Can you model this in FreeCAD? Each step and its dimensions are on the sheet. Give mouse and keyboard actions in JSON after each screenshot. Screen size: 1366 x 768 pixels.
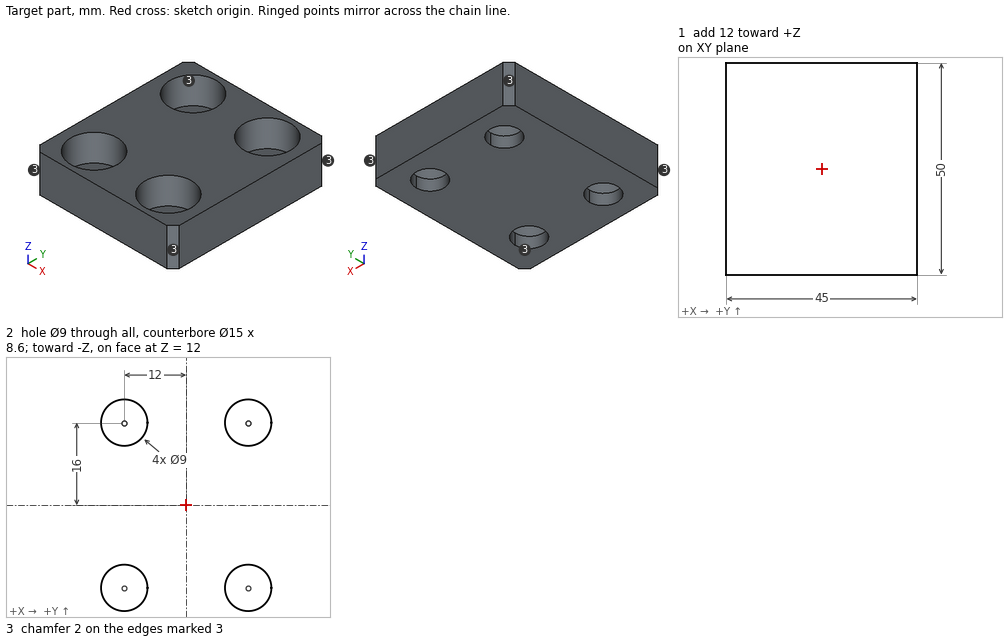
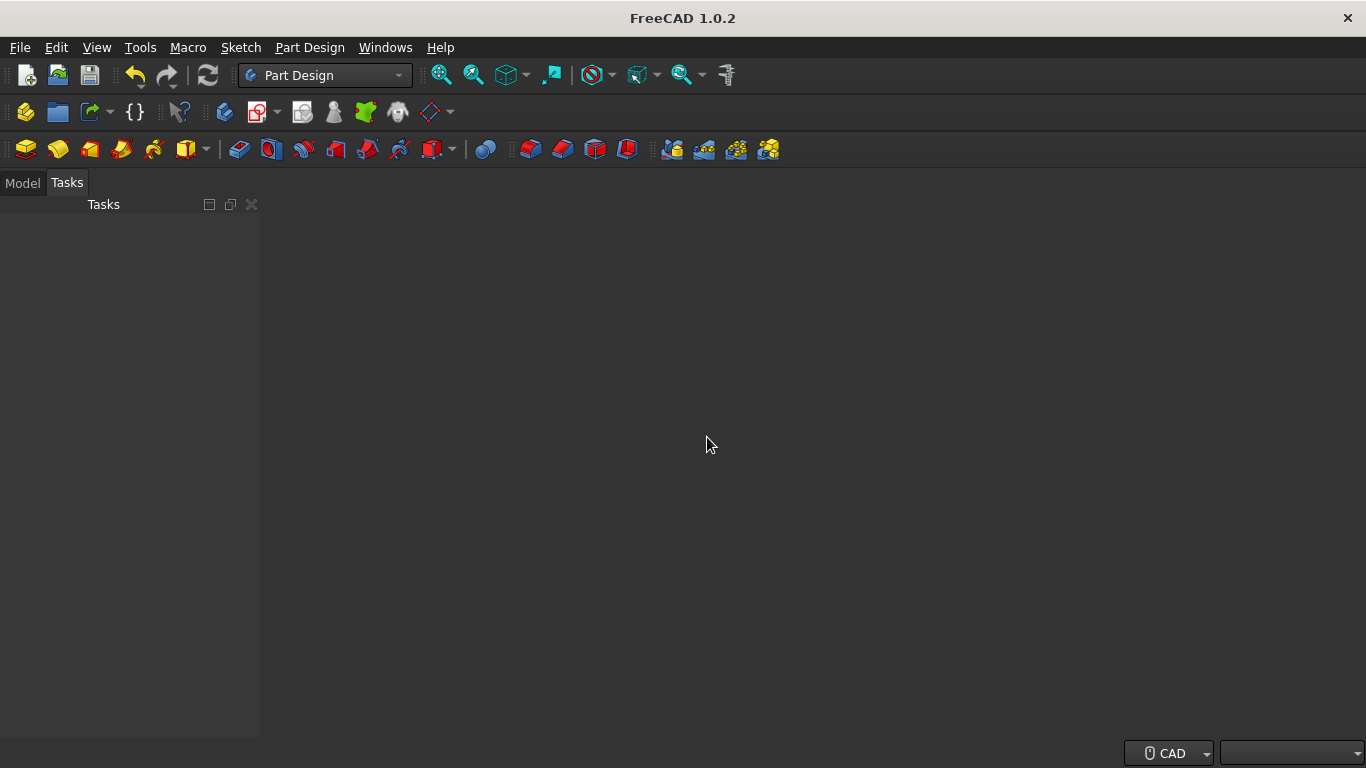
{"action": "left_click", "coordinate": [26, 76]}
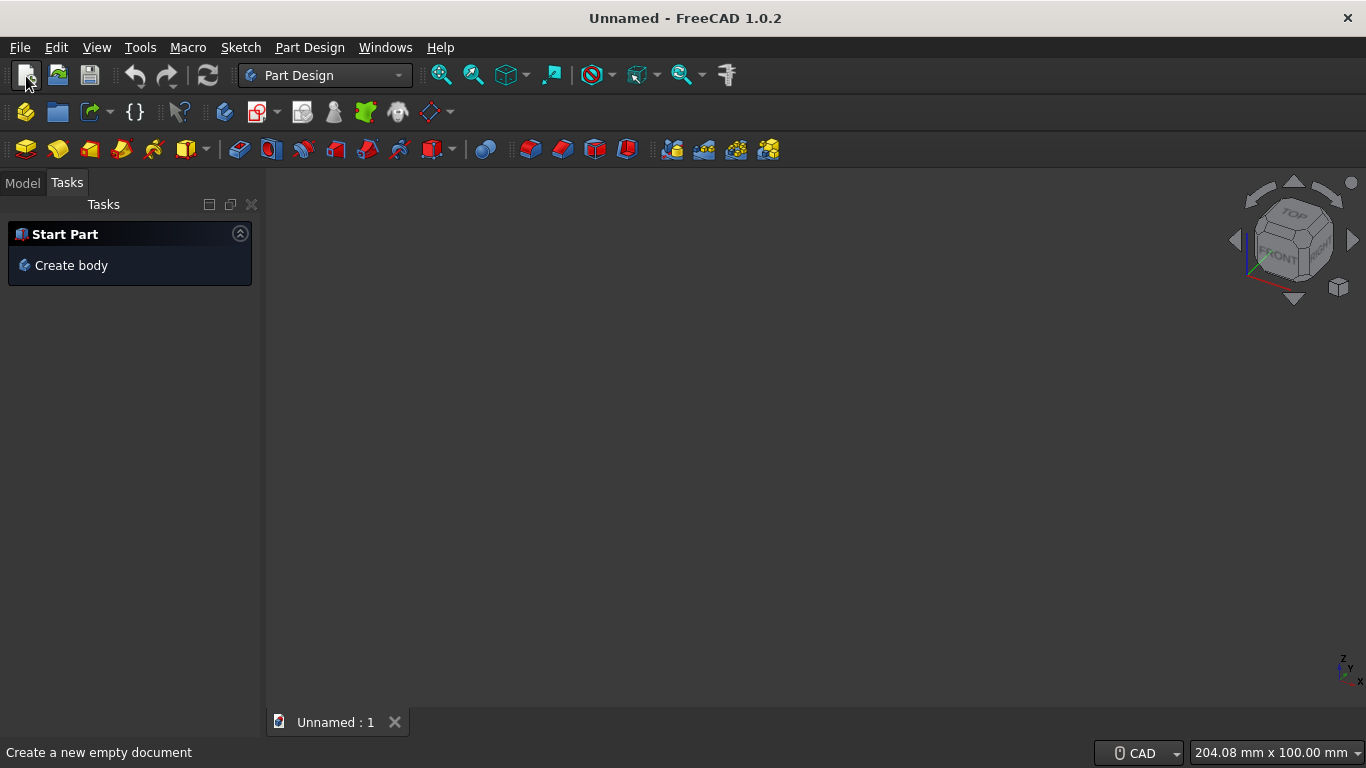
{"action": "left_click", "coordinate": [258, 112]}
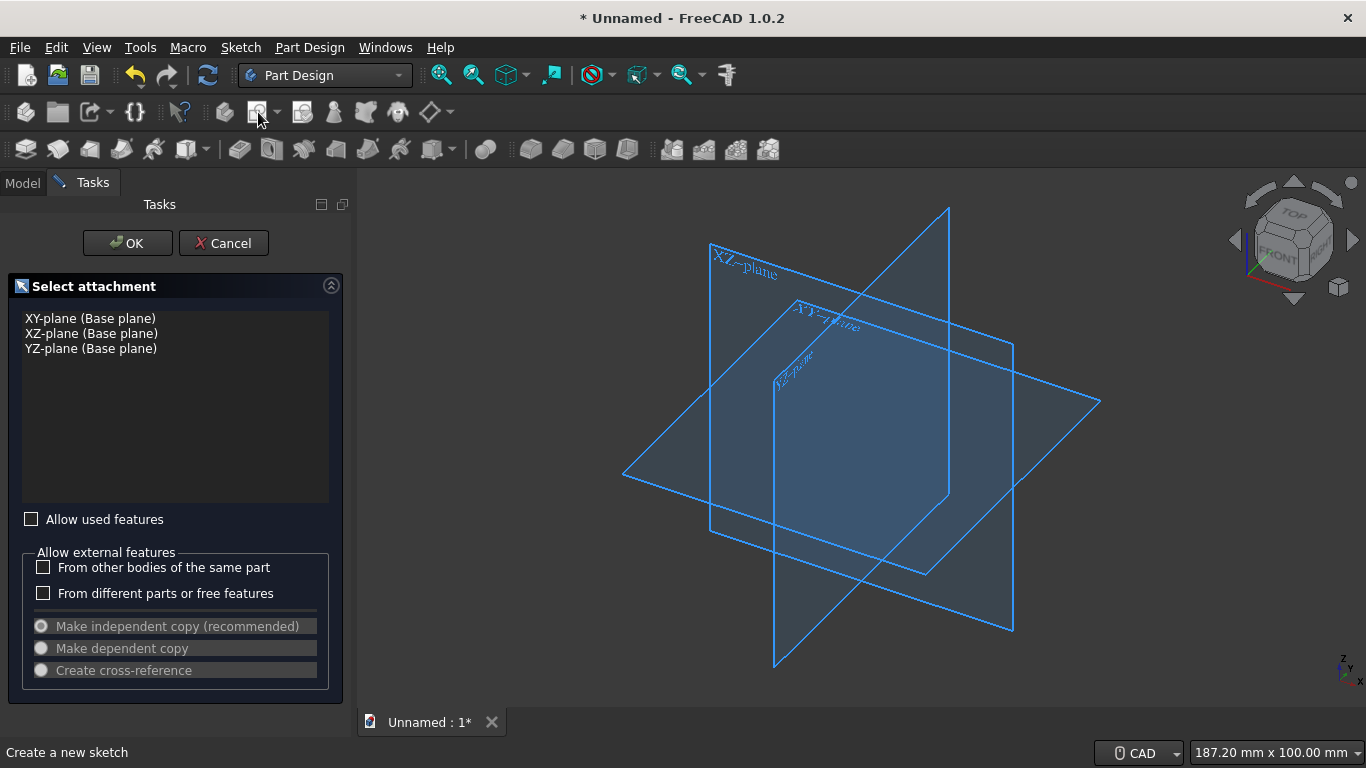
{"action": "left_click", "coordinate": [82, 318]}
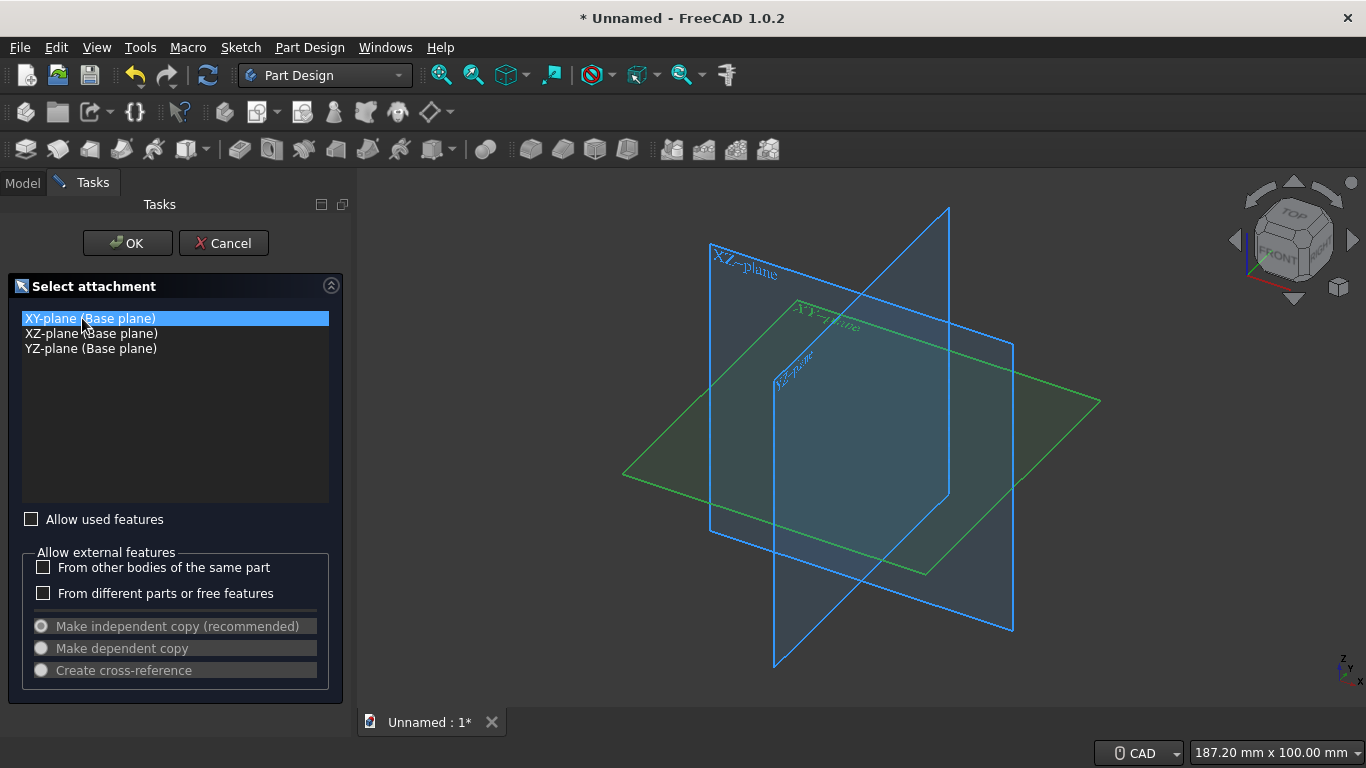
{"action": "left_click", "coordinate": [128, 243]}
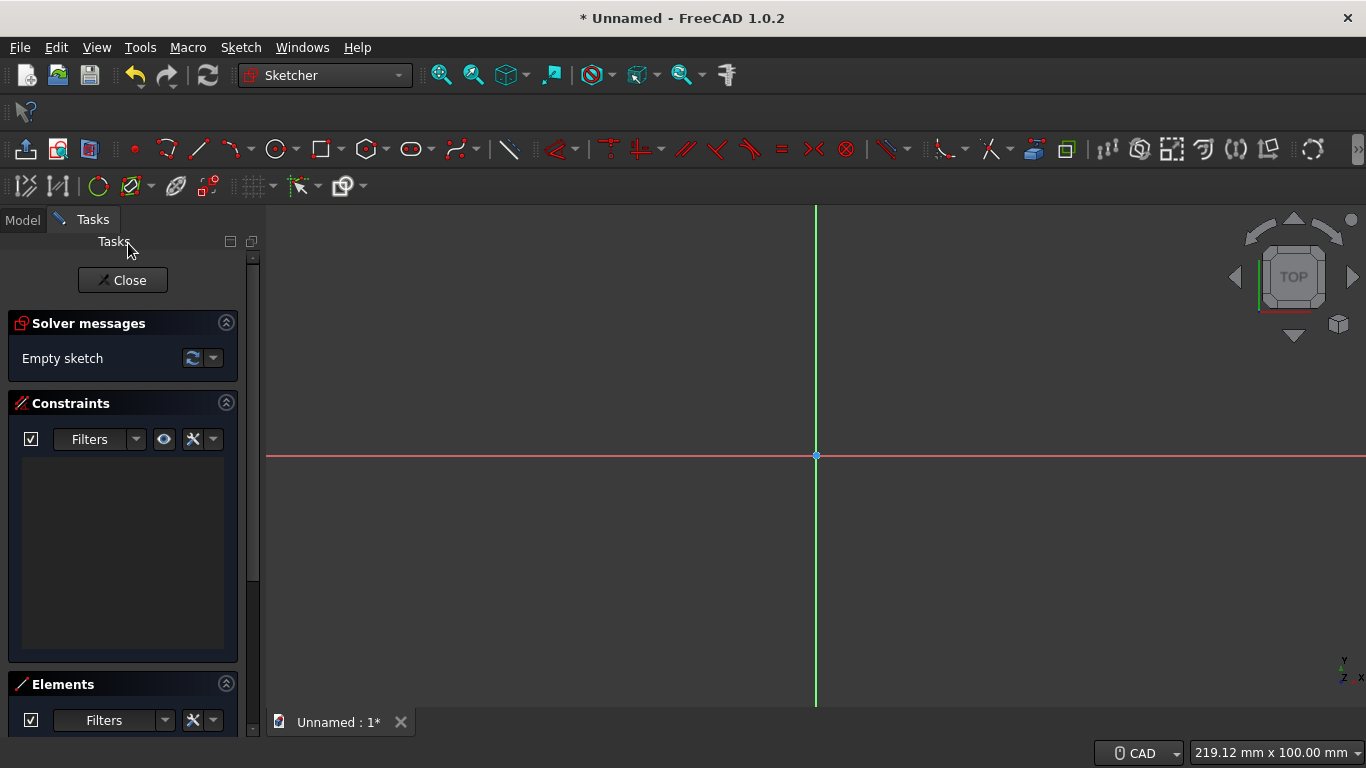
{"action": "key", "text": "g v"}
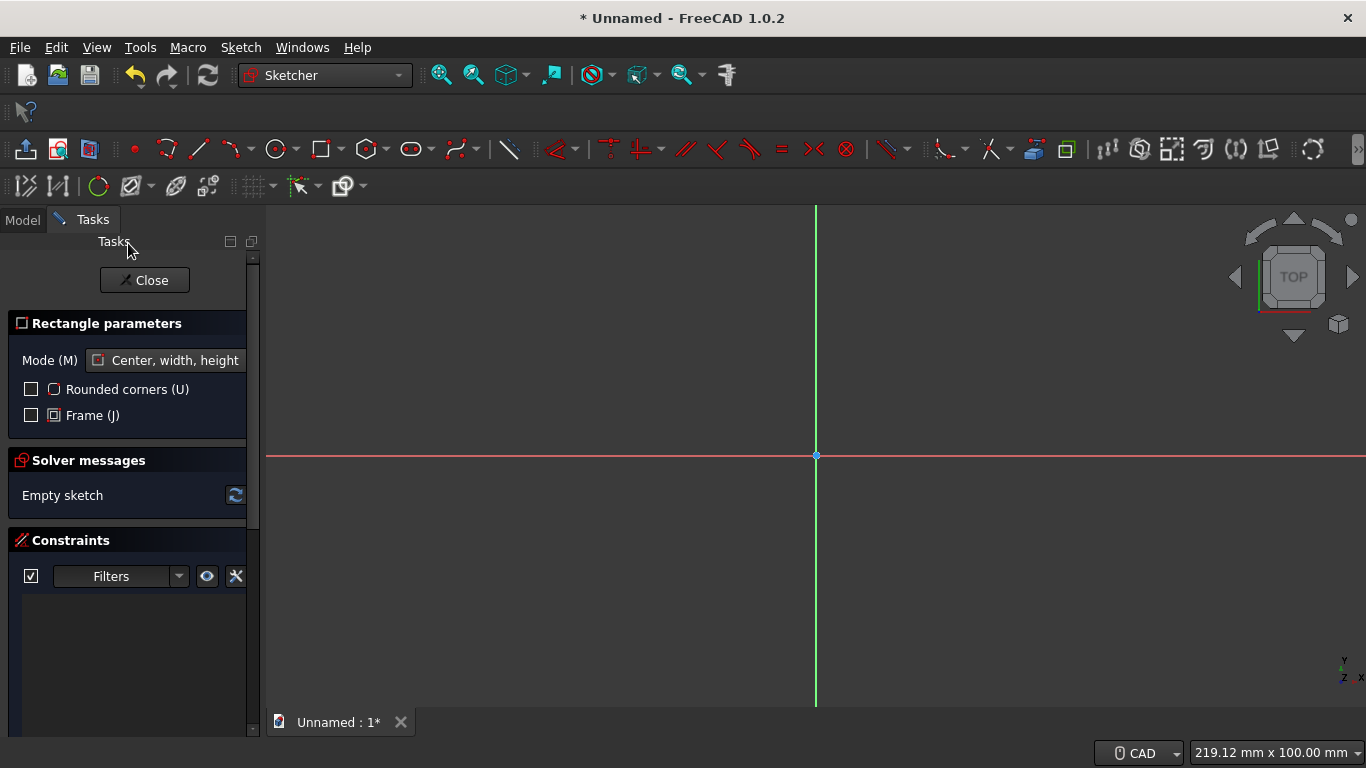
{"action": "left_click", "coordinate": [816, 456]}
{"action": "mouse_move", "coordinate": [929, 330]}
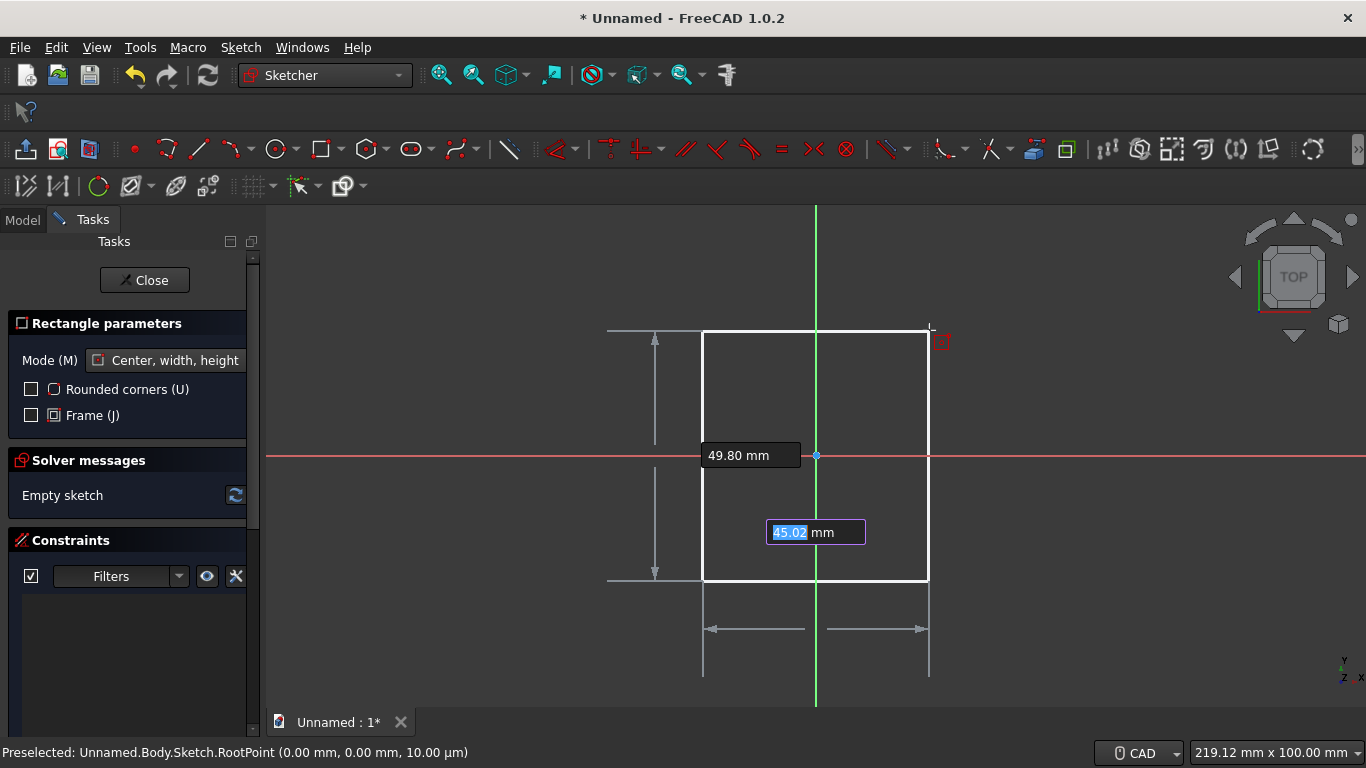
{"action": "type", "text": "45"}
{"action": "key", "text": "Tab"}
{"action": "type", "text": "50"}
{"action": "key", "text": "Return"}
{"action": "key", "text": "Escape"}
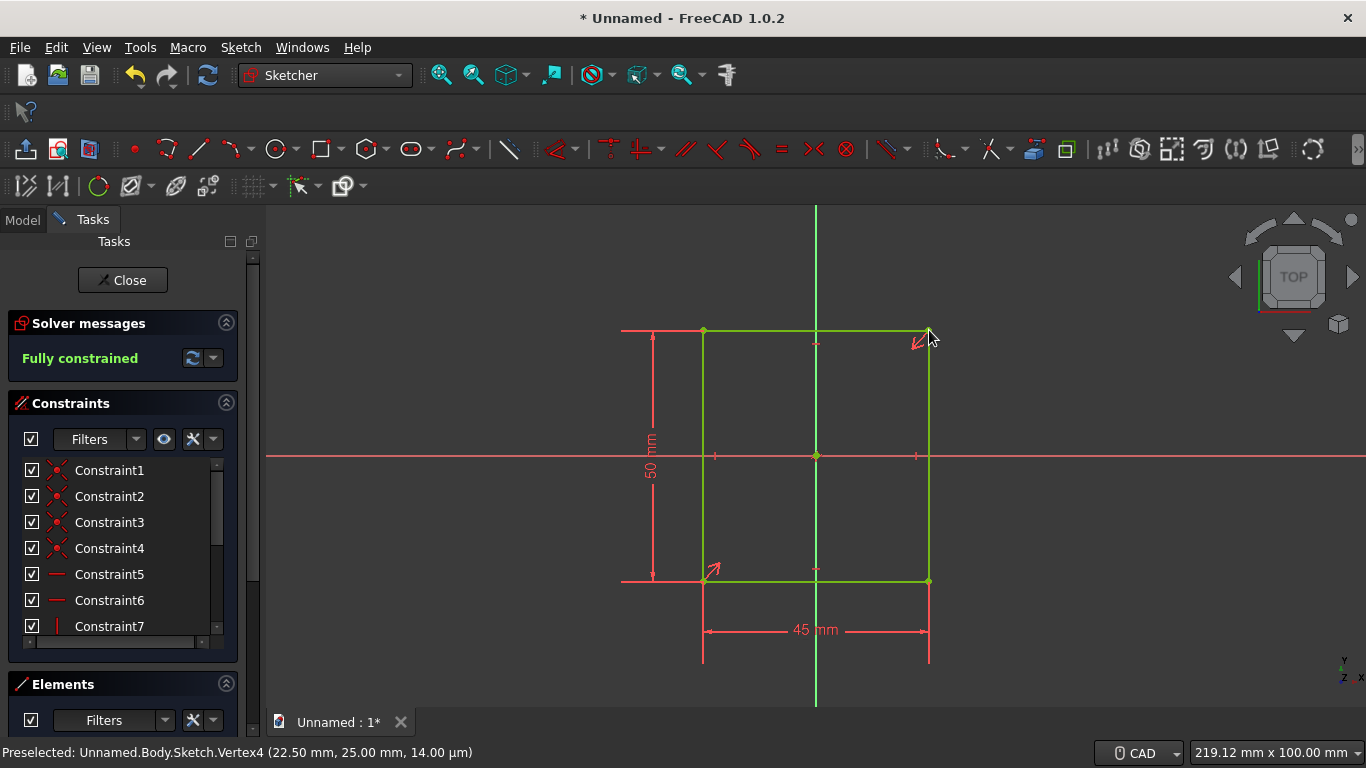
{"action": "left_click", "coordinate": [123, 280]}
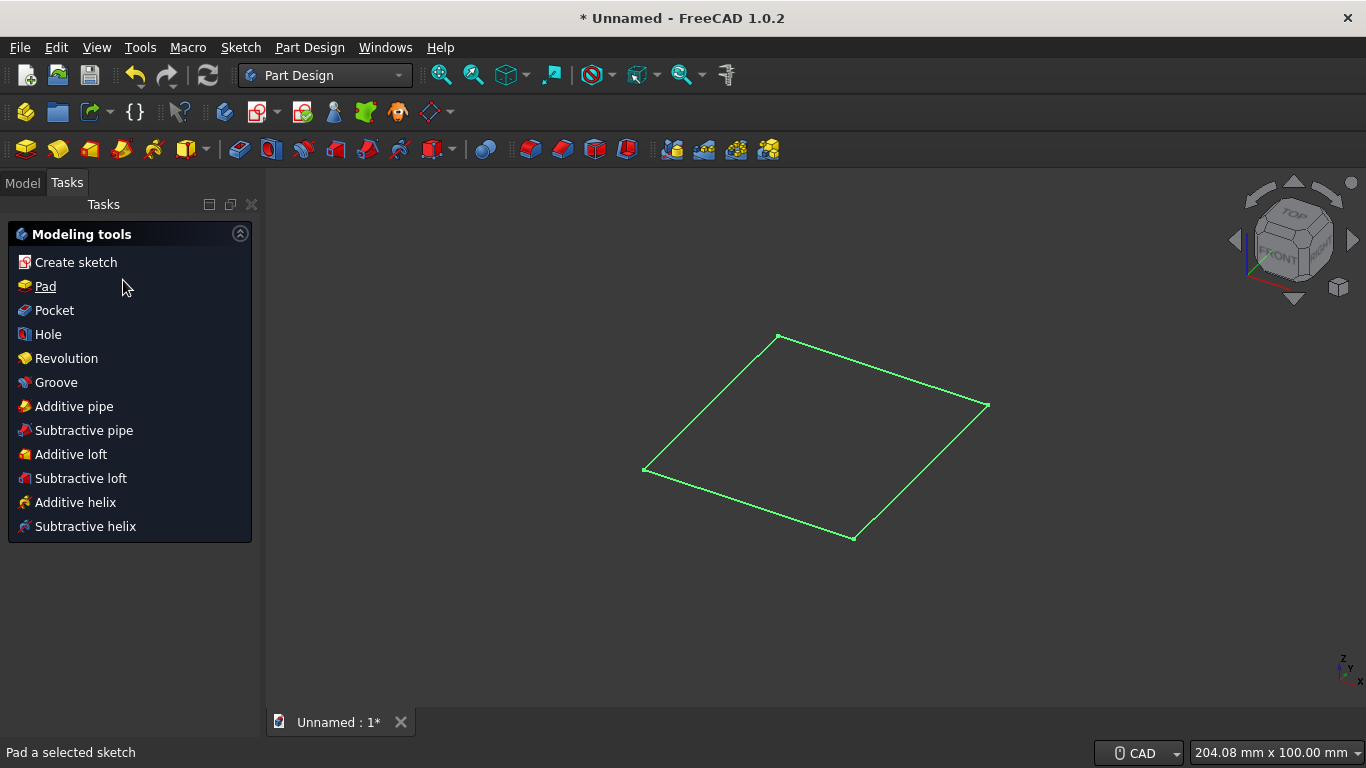
{"action": "left_click", "coordinate": [26, 150]}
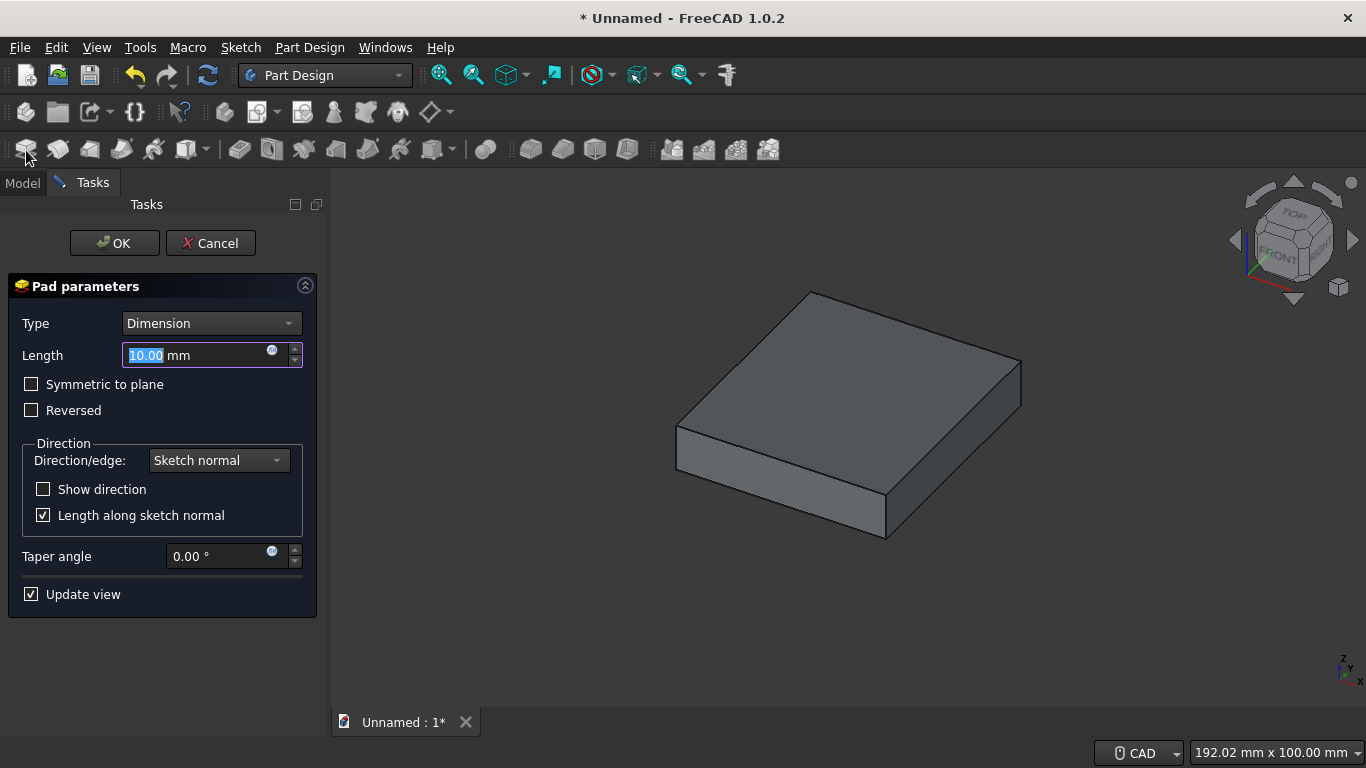
{"action": "type", "text": "12"}
{"action": "key", "text": "Tab"}